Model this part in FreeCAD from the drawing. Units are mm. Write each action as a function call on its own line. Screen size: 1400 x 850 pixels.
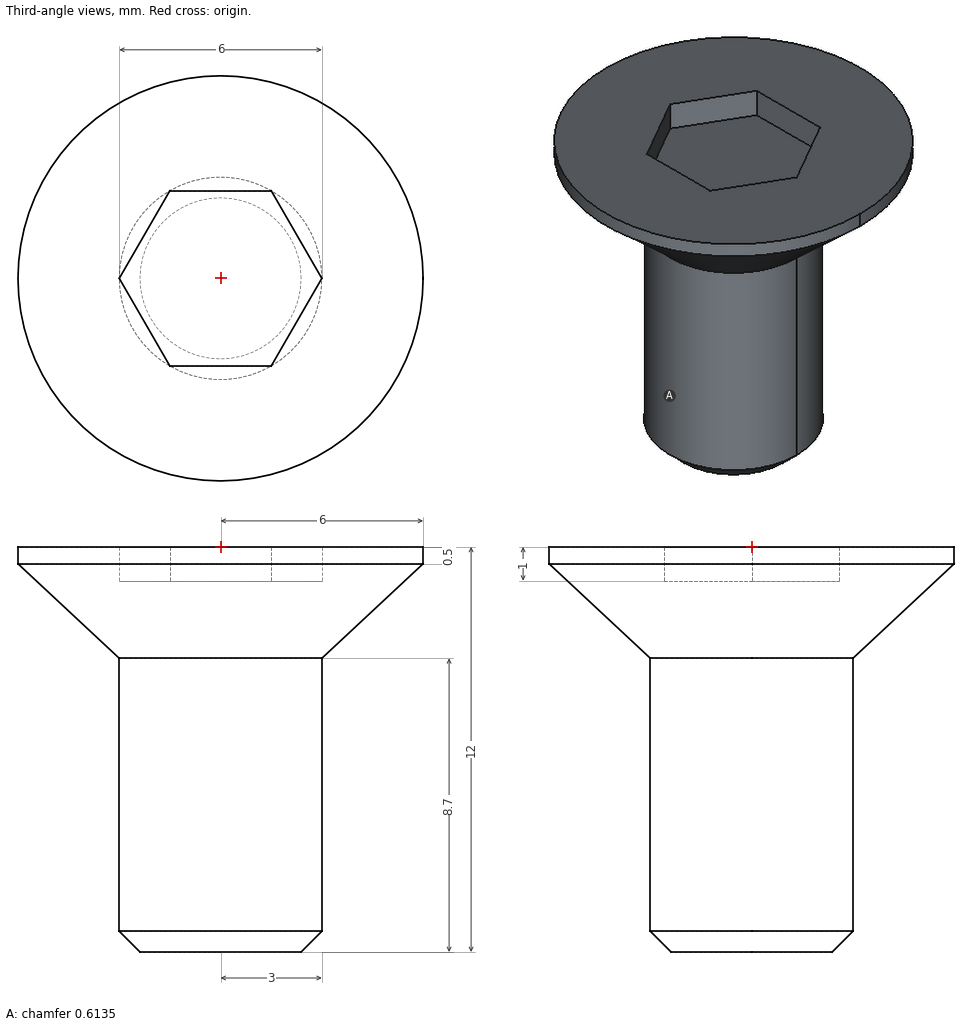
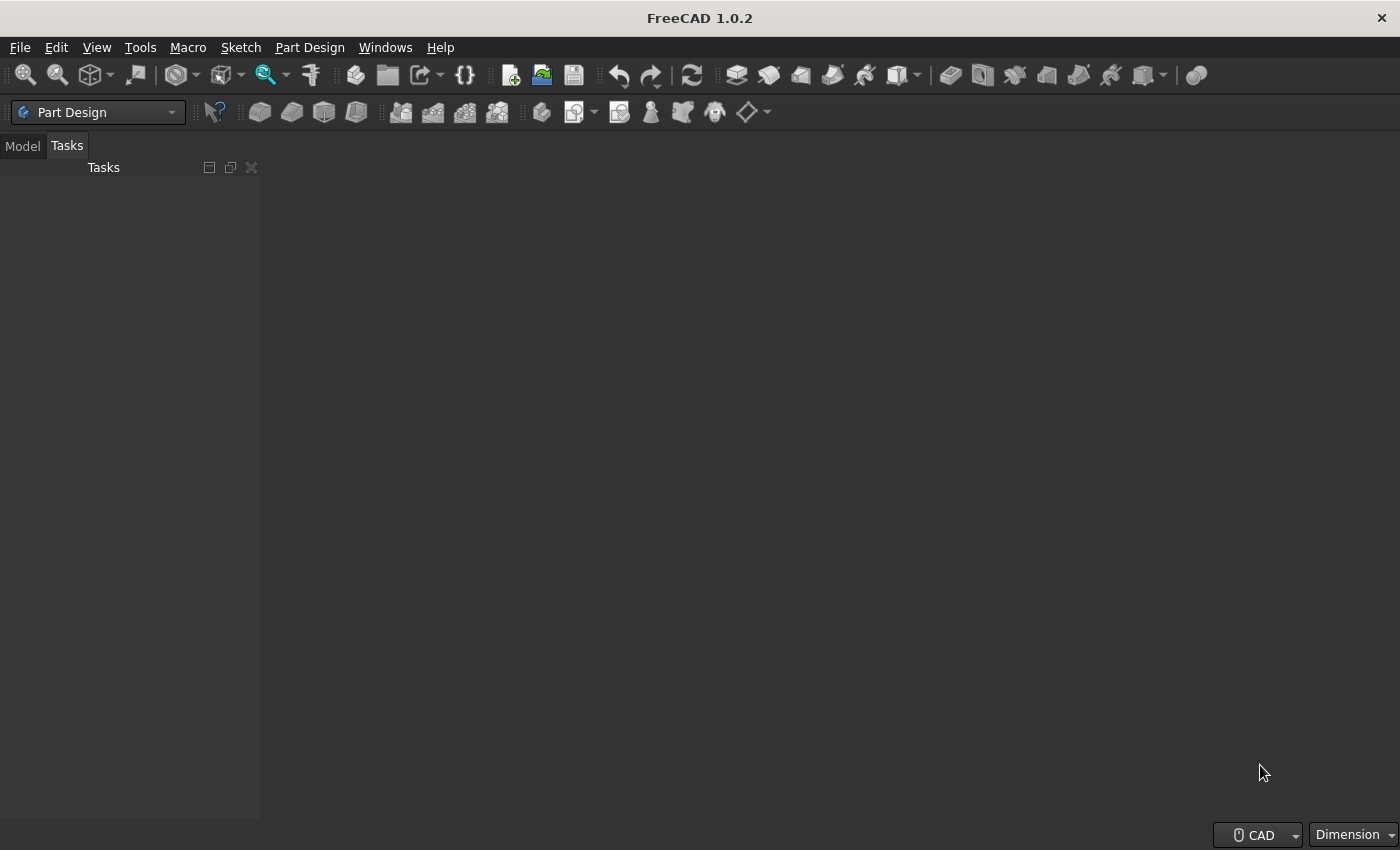
key(ctrl+n)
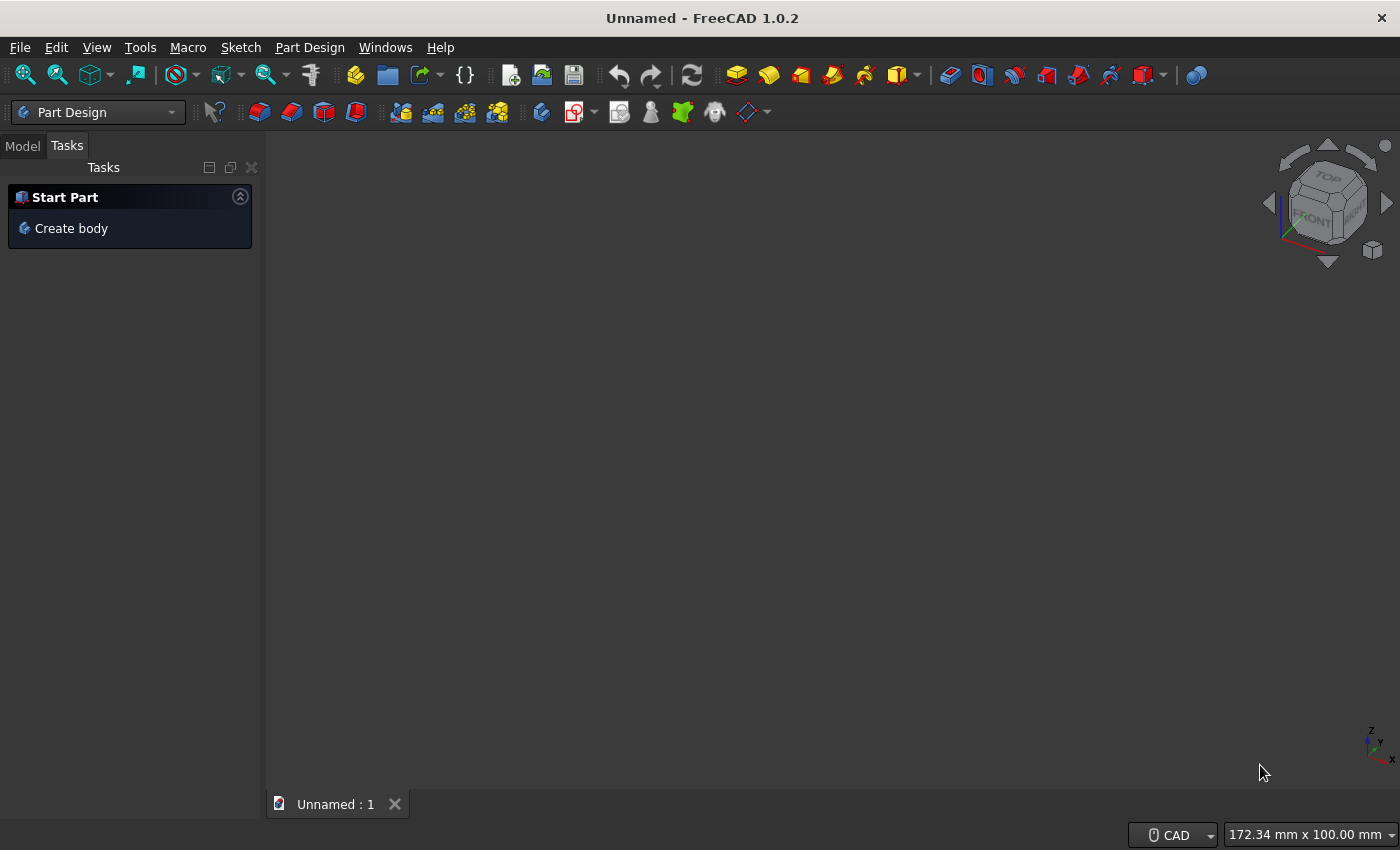
click(574, 112)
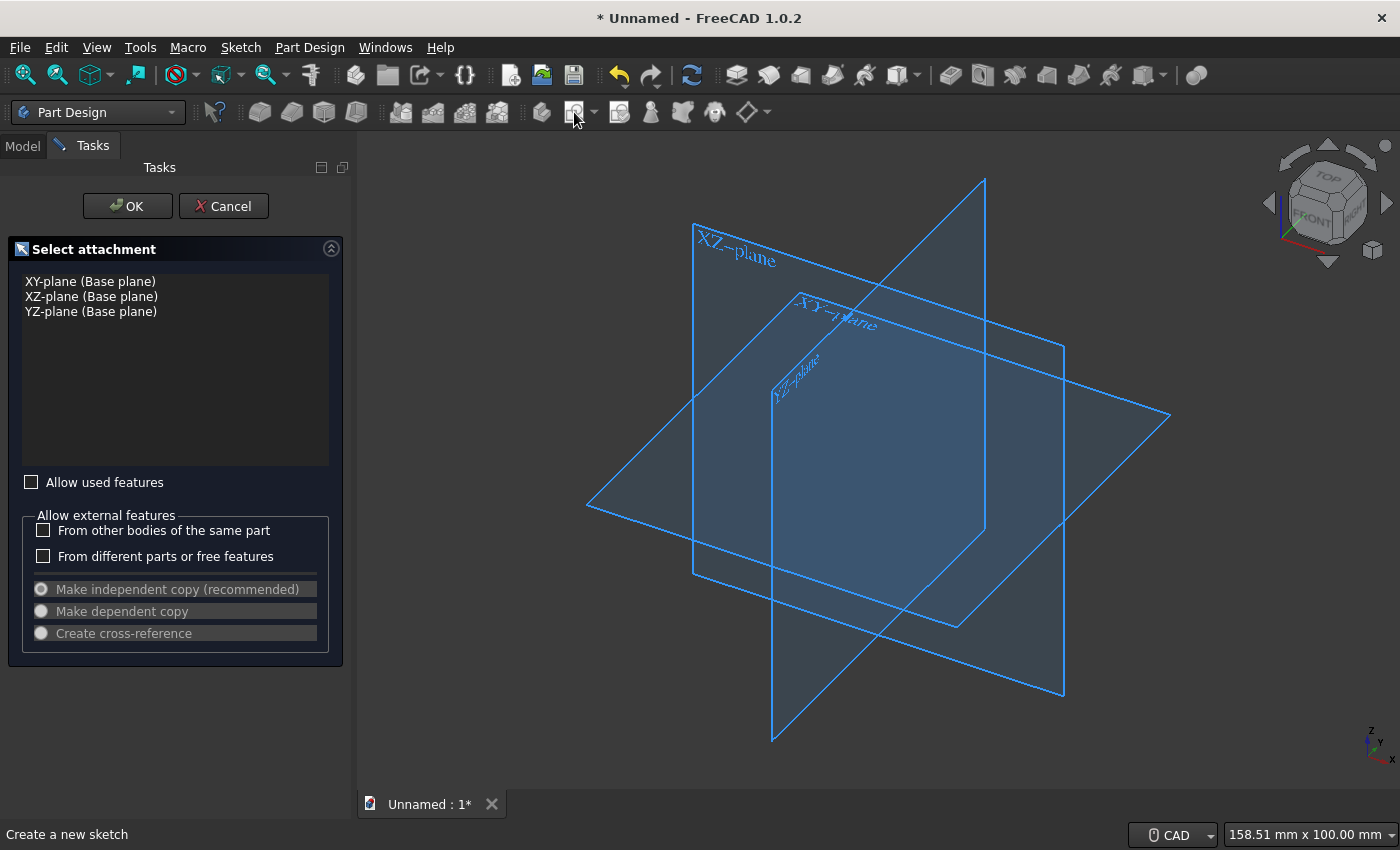
click(82, 296)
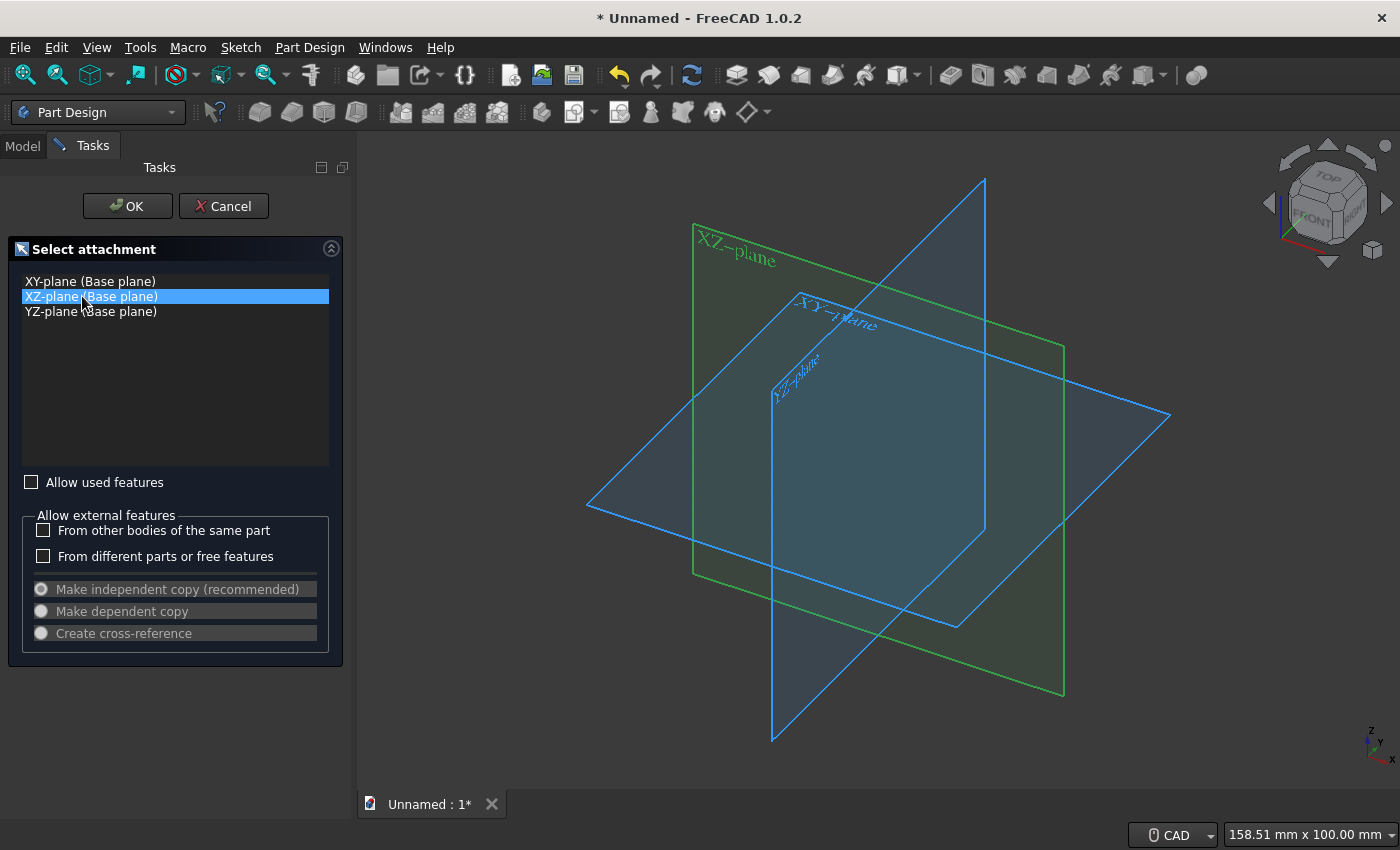
click(128, 206)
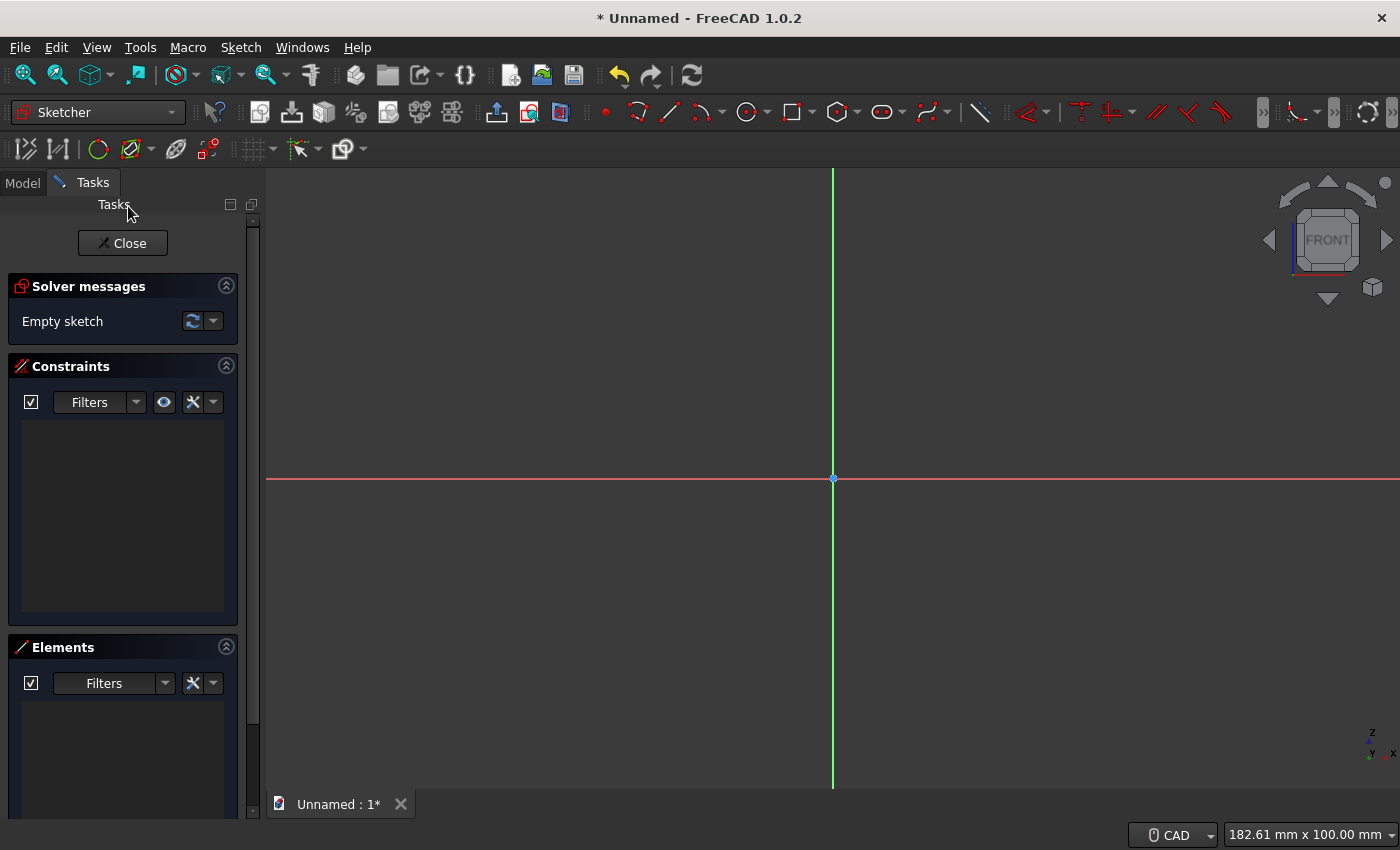
scroll(874, 525, up, 8)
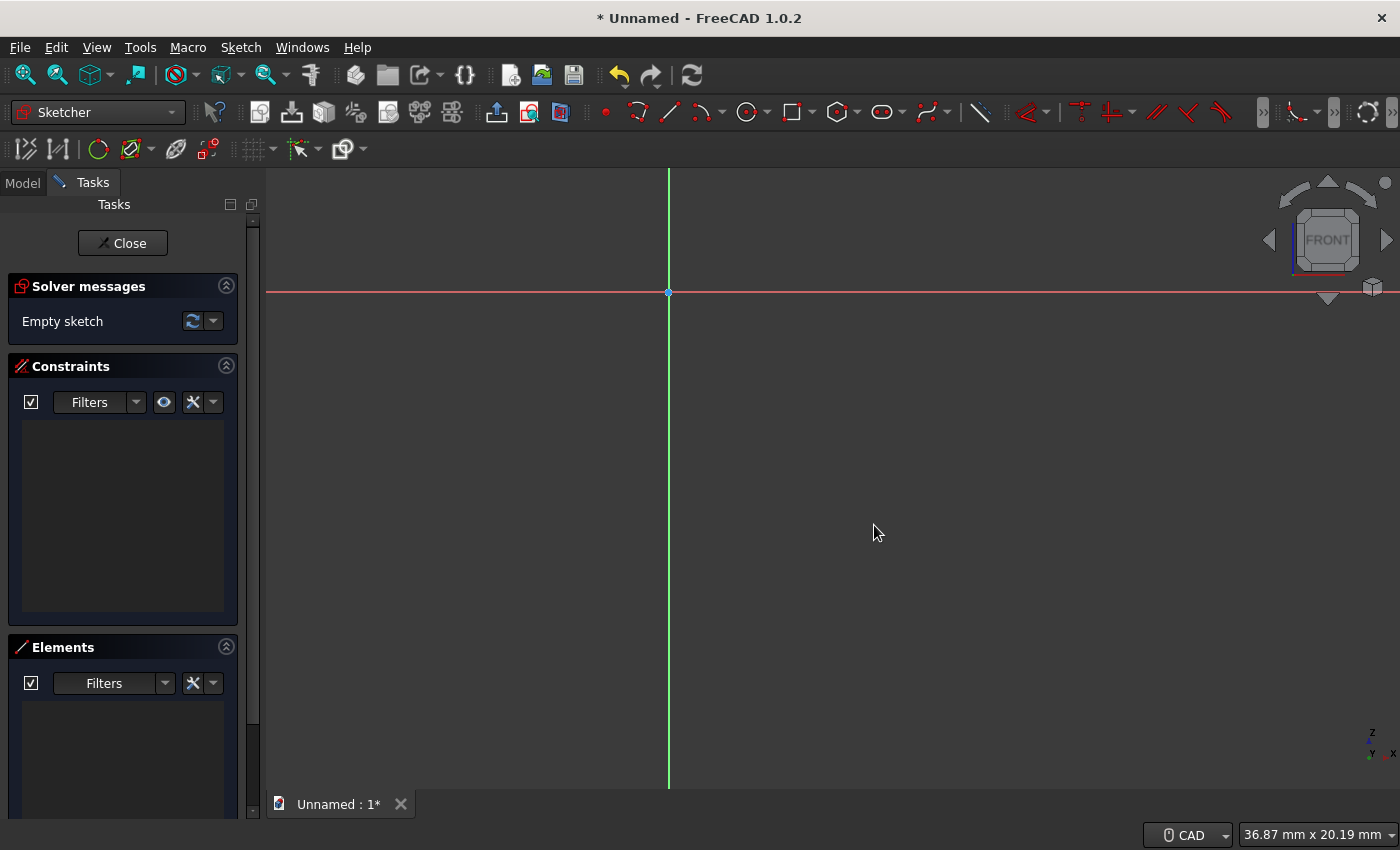
key(g)
key(m)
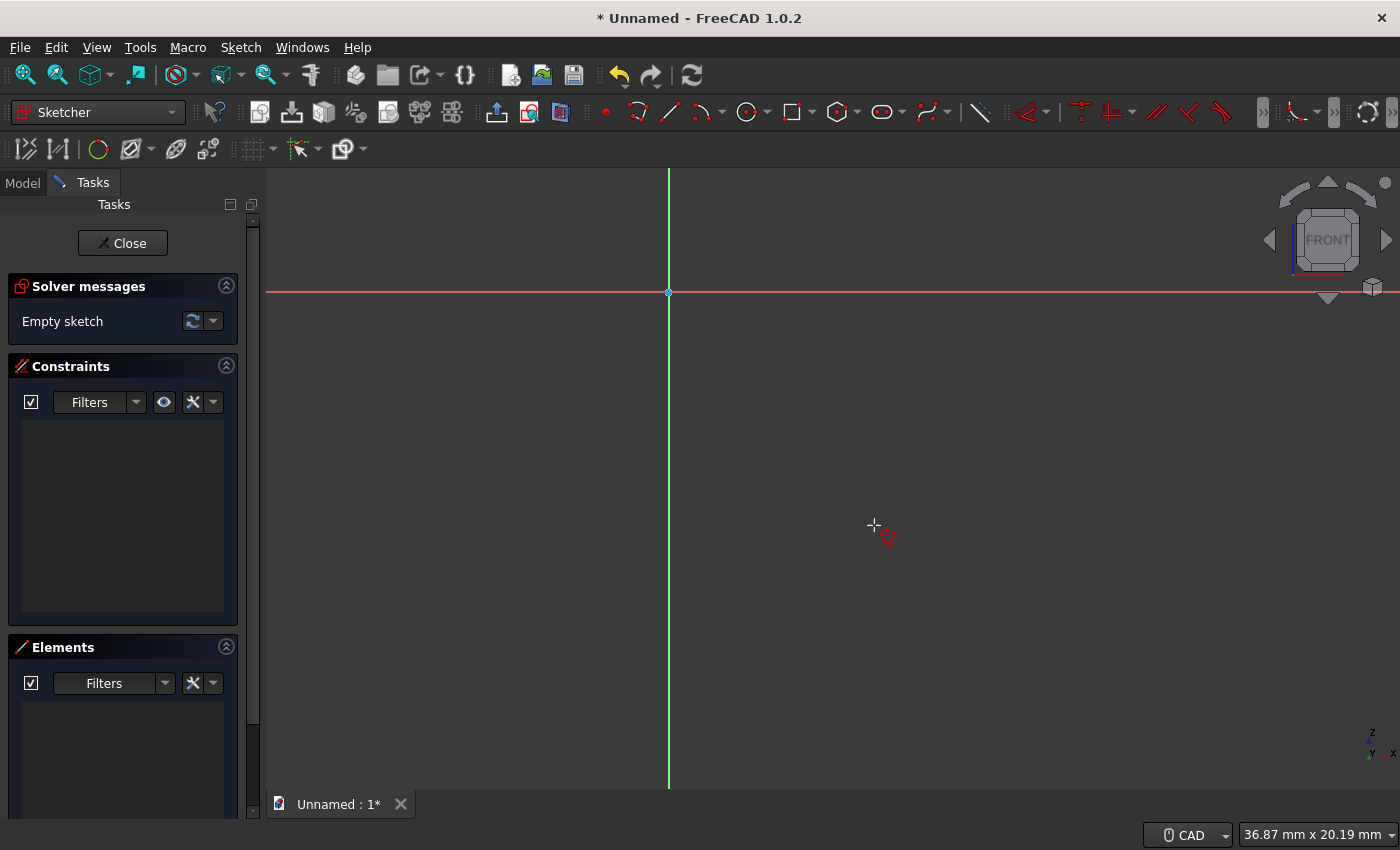
click(669, 292)
click(853, 301)
click(853, 308)
click(761, 394)
click(761, 662)
click(678, 662)
click(669, 292)
key(Escape)
key(Escape)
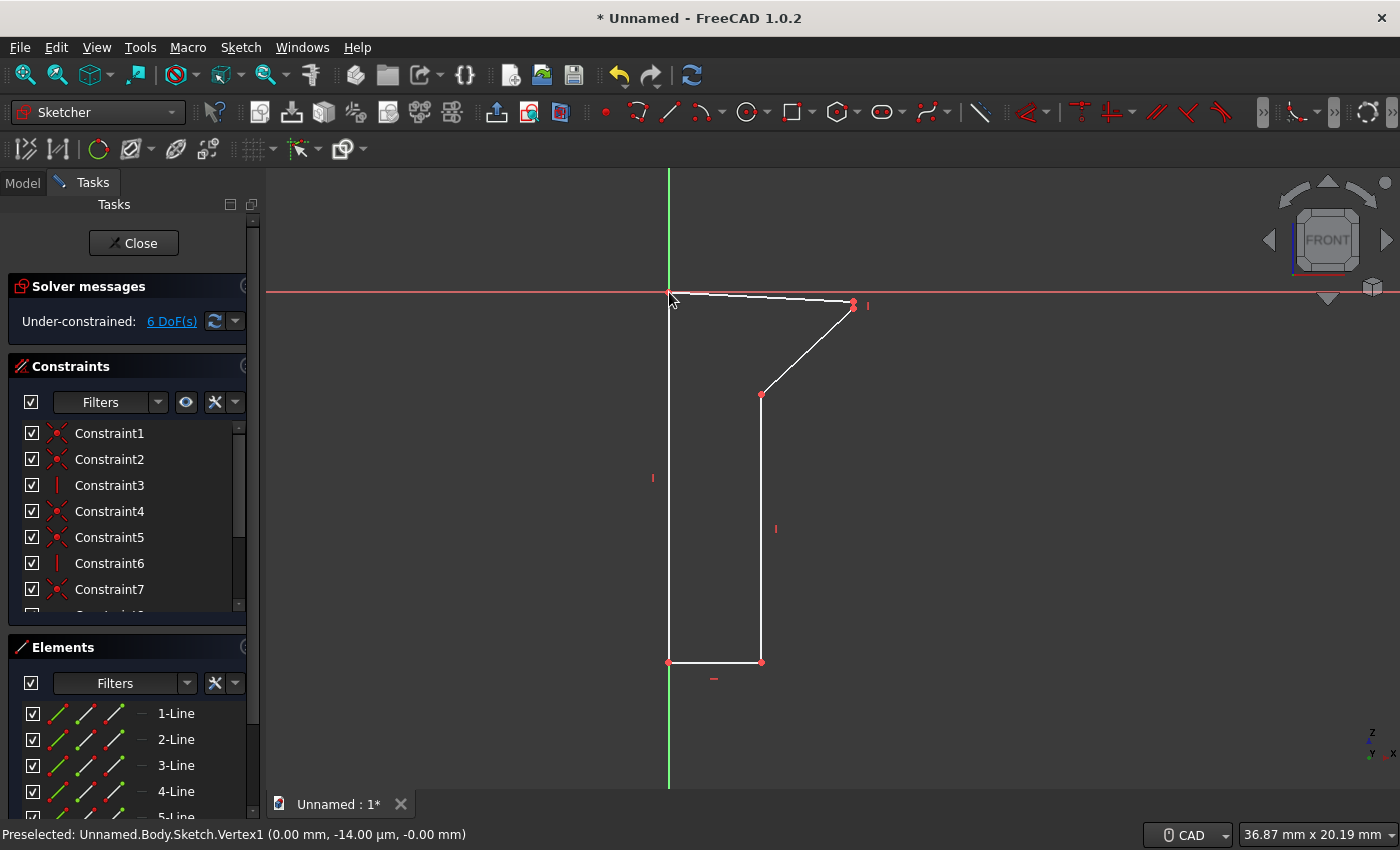
click(724, 295)